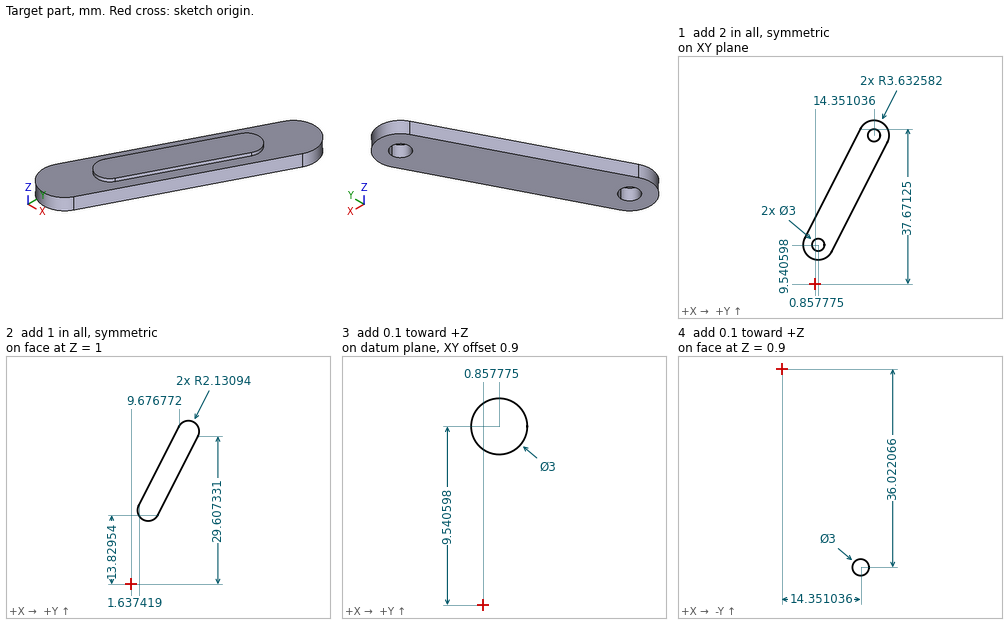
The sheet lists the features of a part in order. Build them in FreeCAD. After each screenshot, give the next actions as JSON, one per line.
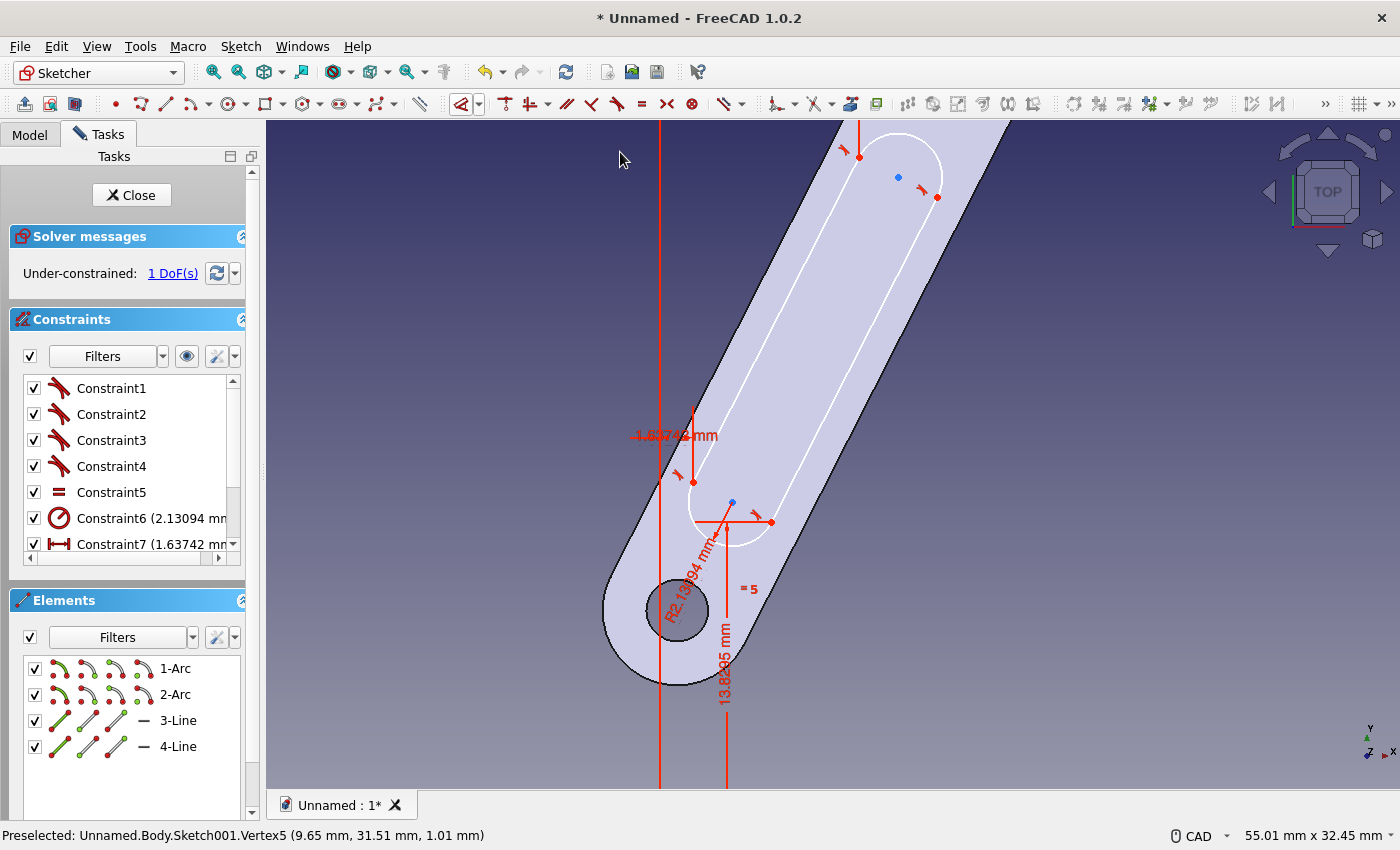
{"action": "left_click", "coordinate": [937, 197]}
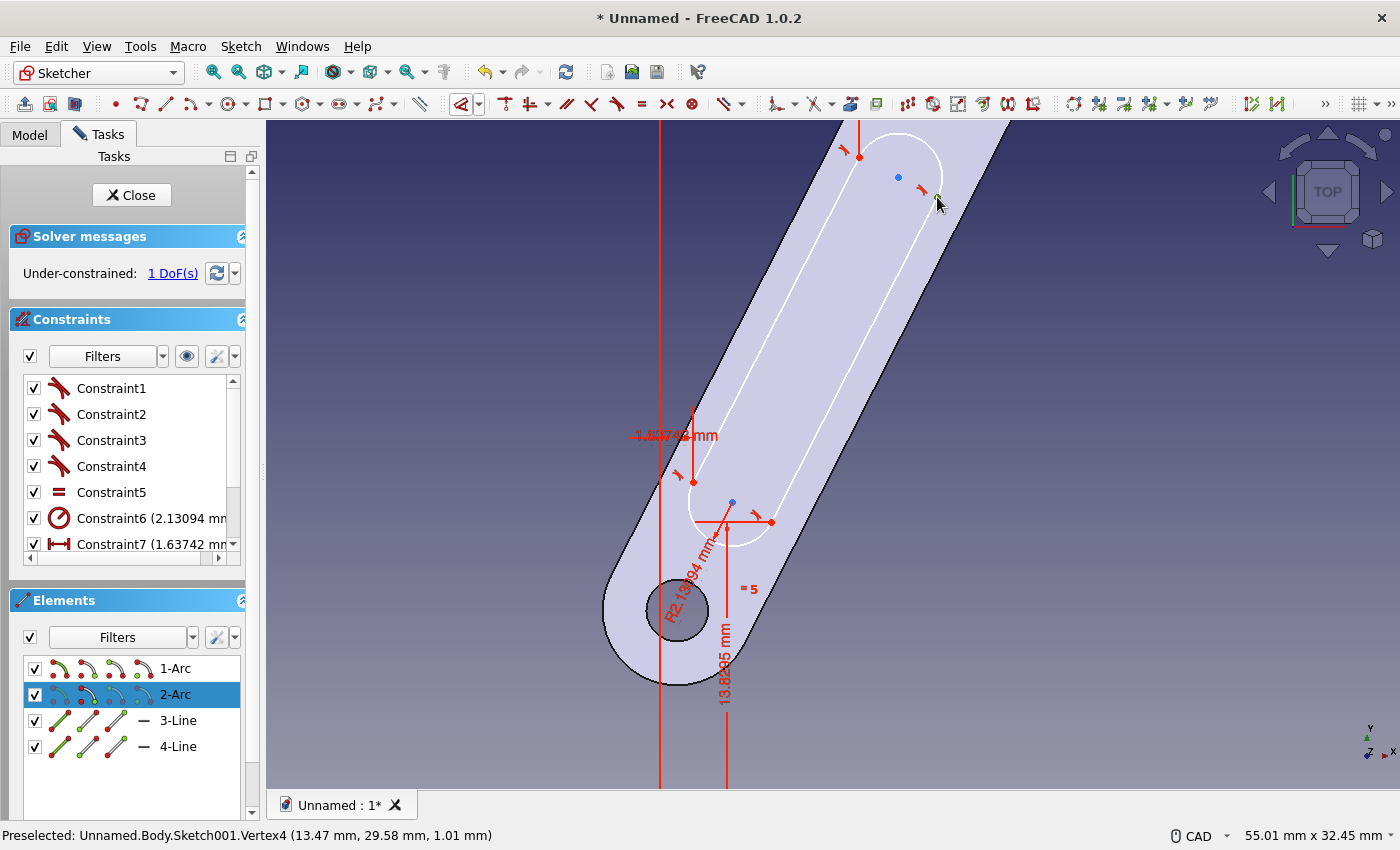
{"action": "key", "text": "i"}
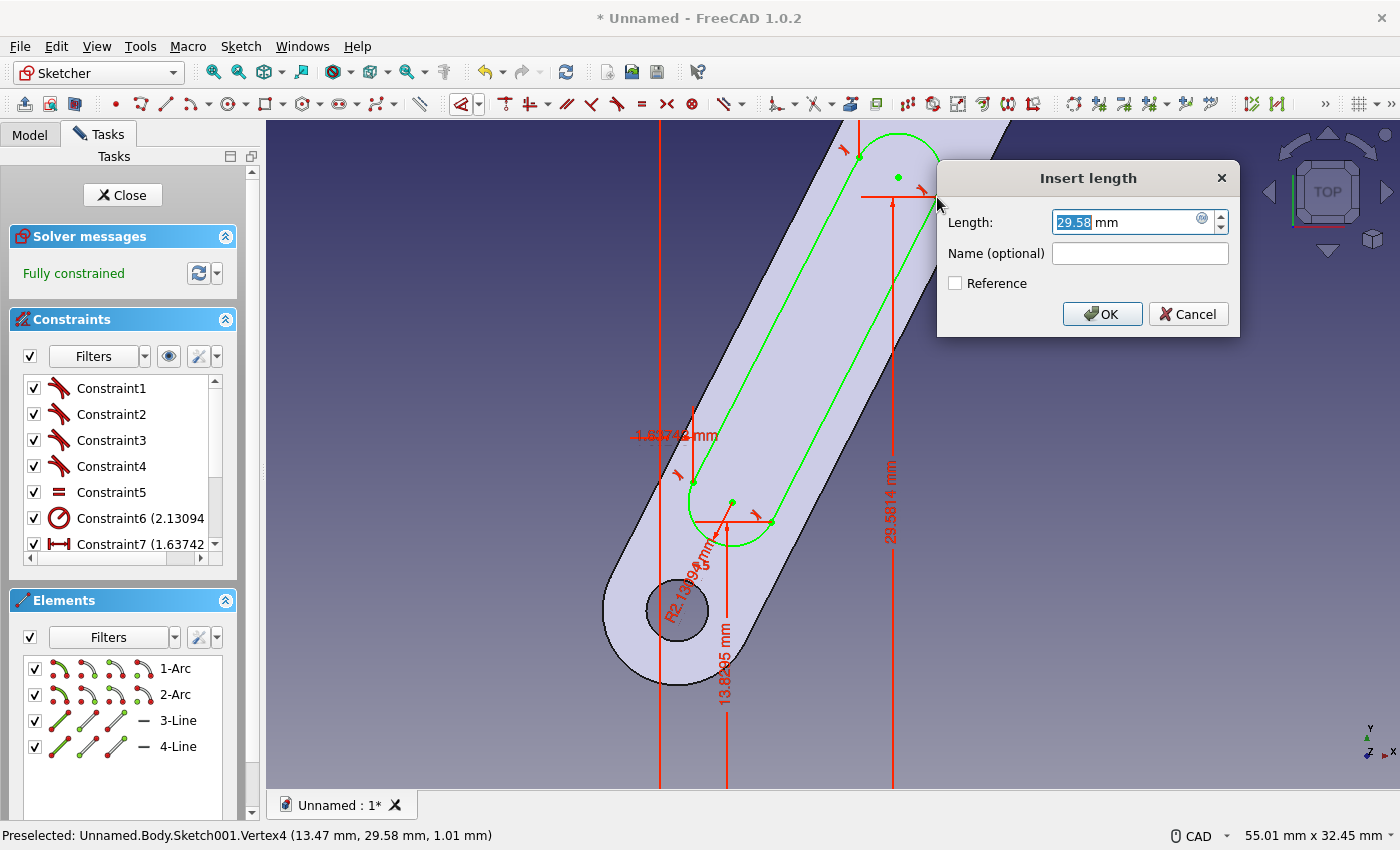
{"action": "type", "text": "29.607331"}
{"action": "key", "text": "Return"}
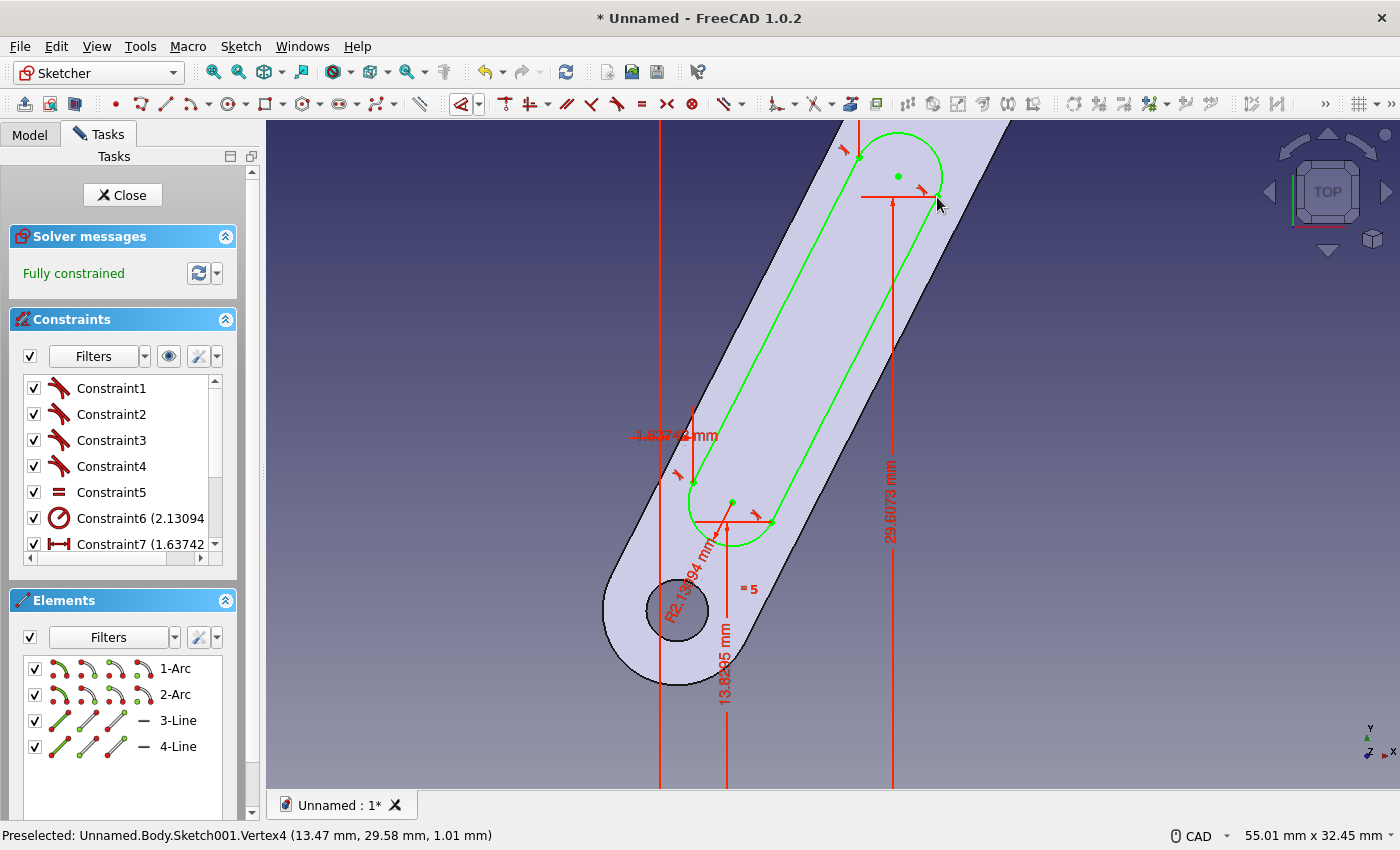
{"action": "left_click", "coordinate": [123, 195]}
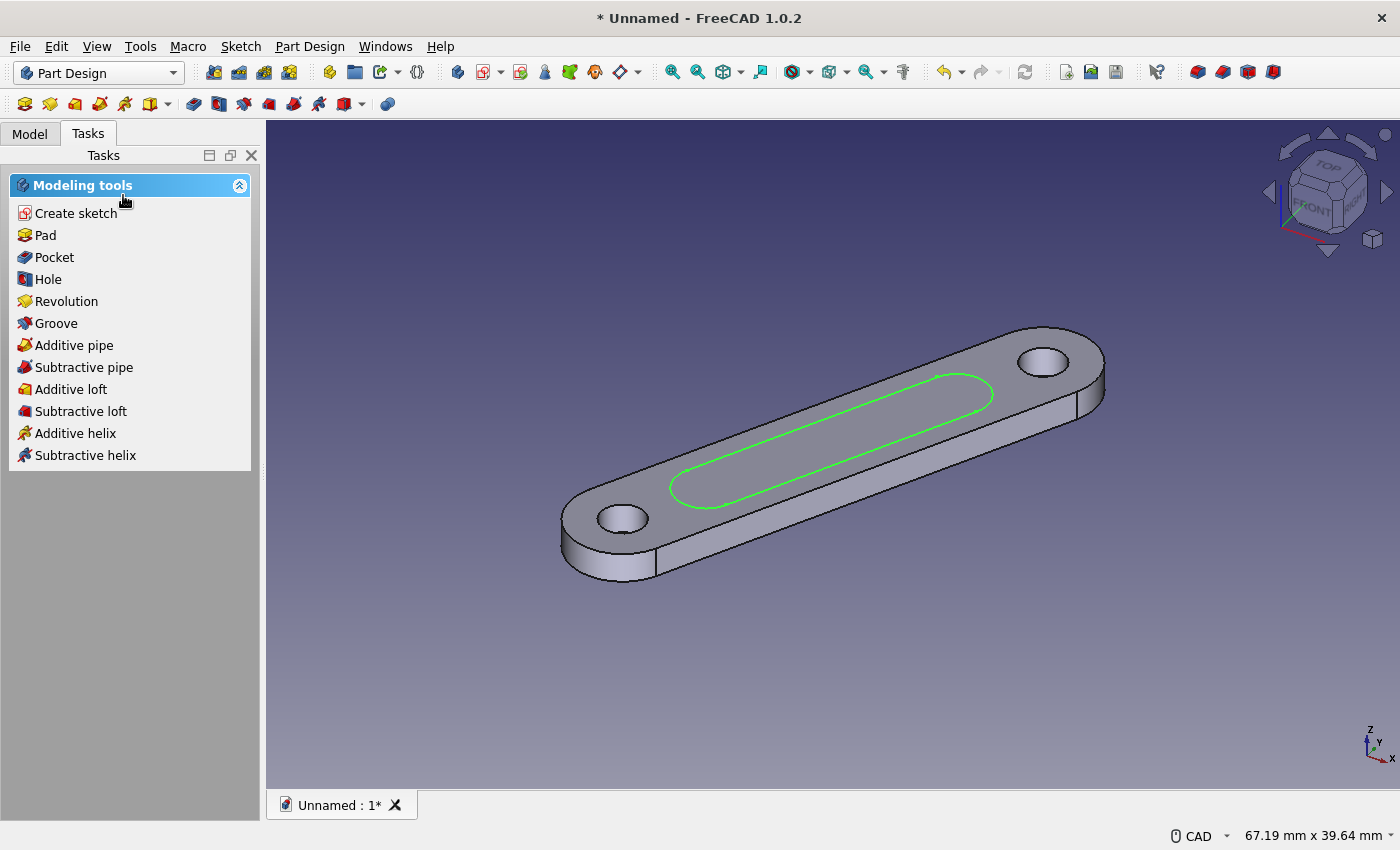
{"action": "left_click", "coordinate": [25, 104]}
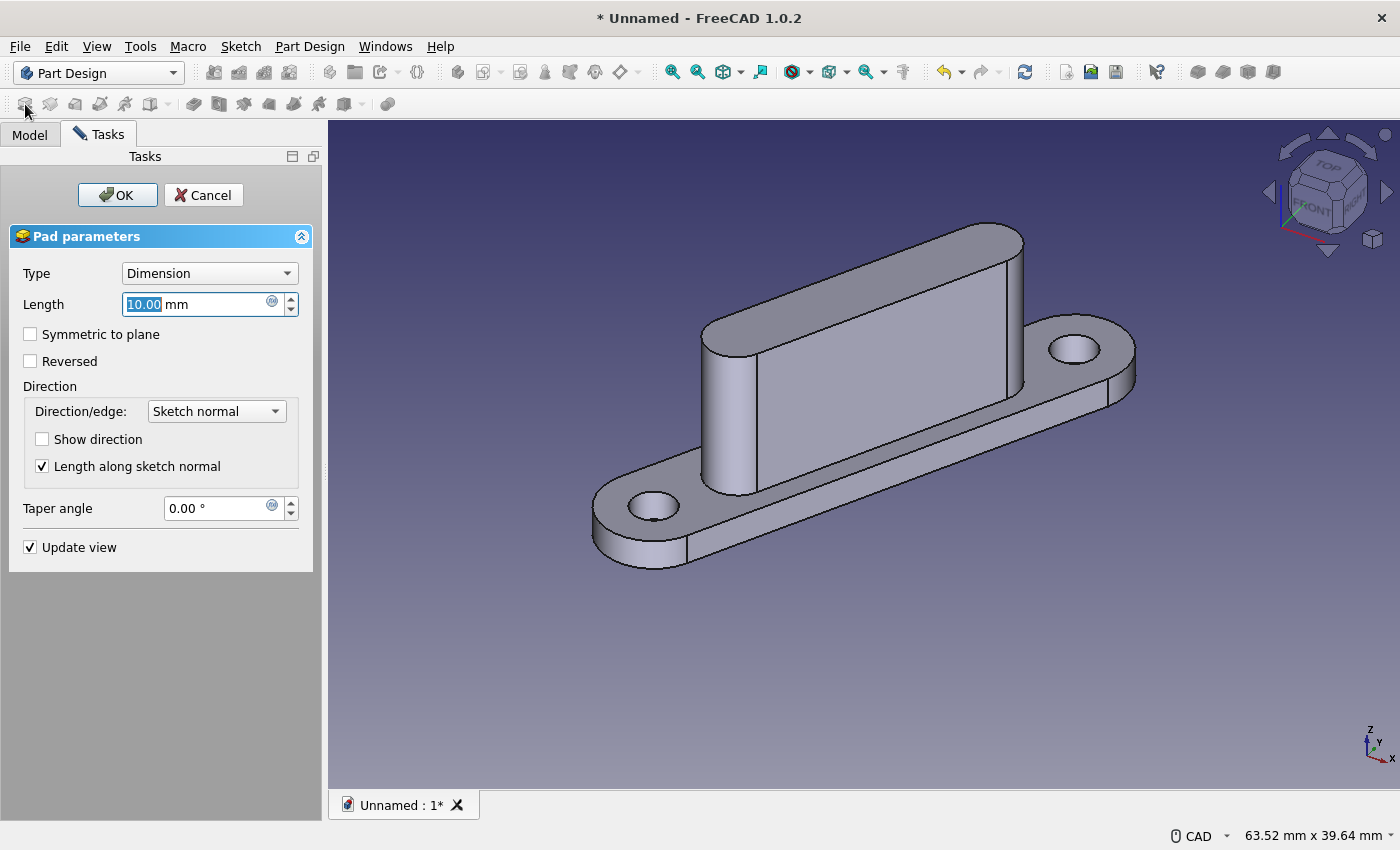
{"action": "type", "text": "1"}
{"action": "key", "text": "Tab"}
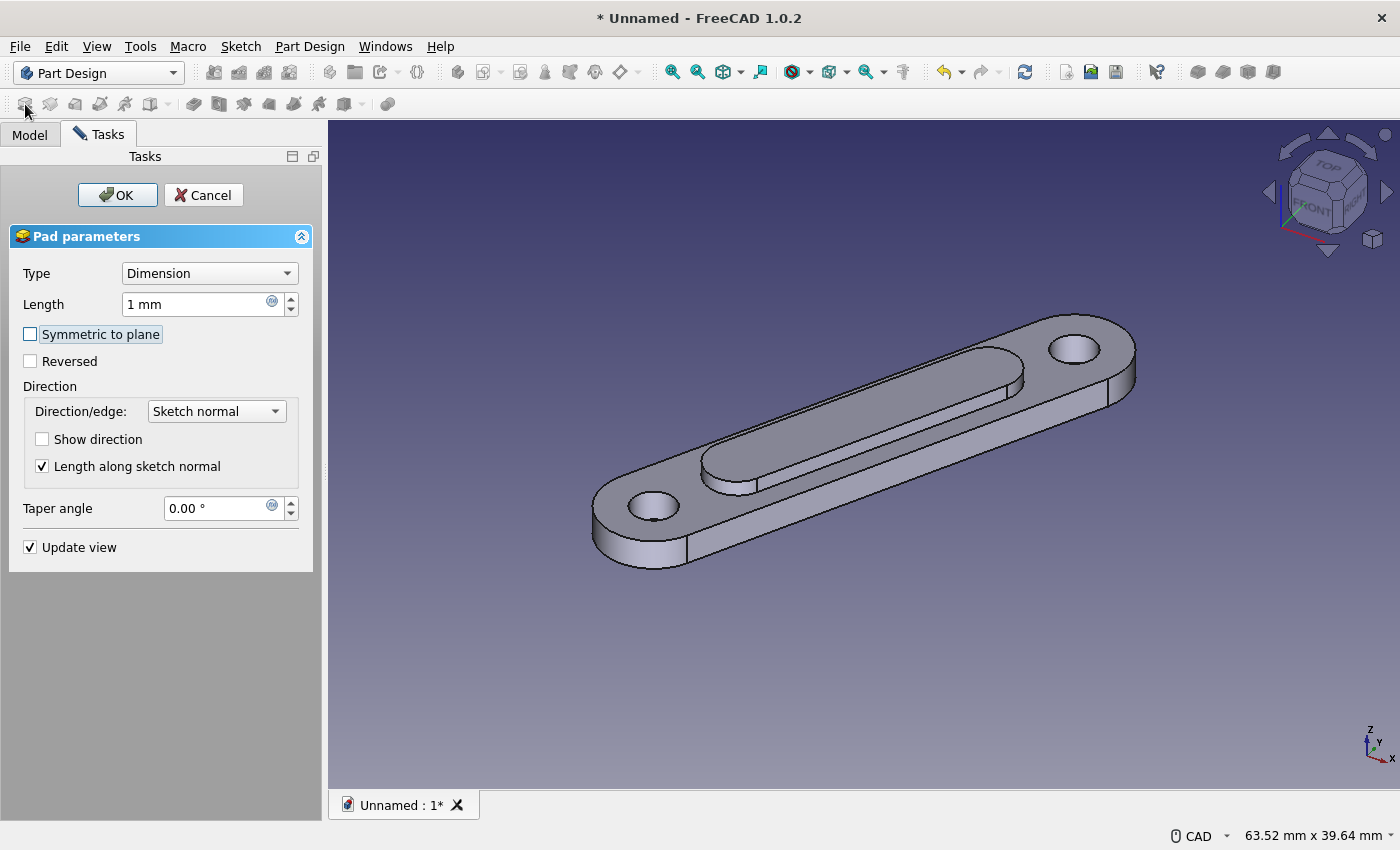
{"action": "left_click", "coordinate": [31, 334]}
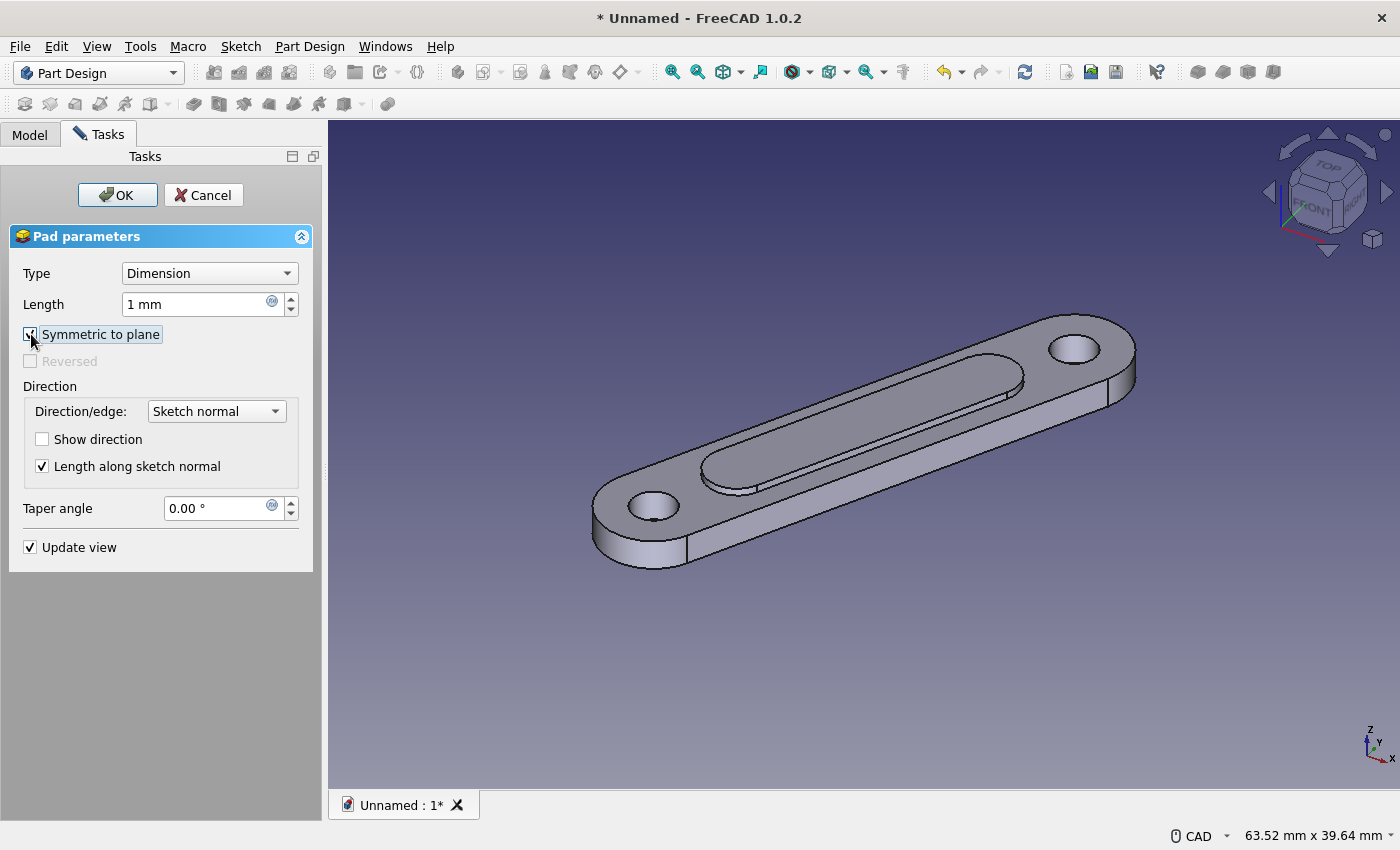
{"action": "left_click", "coordinate": [118, 195]}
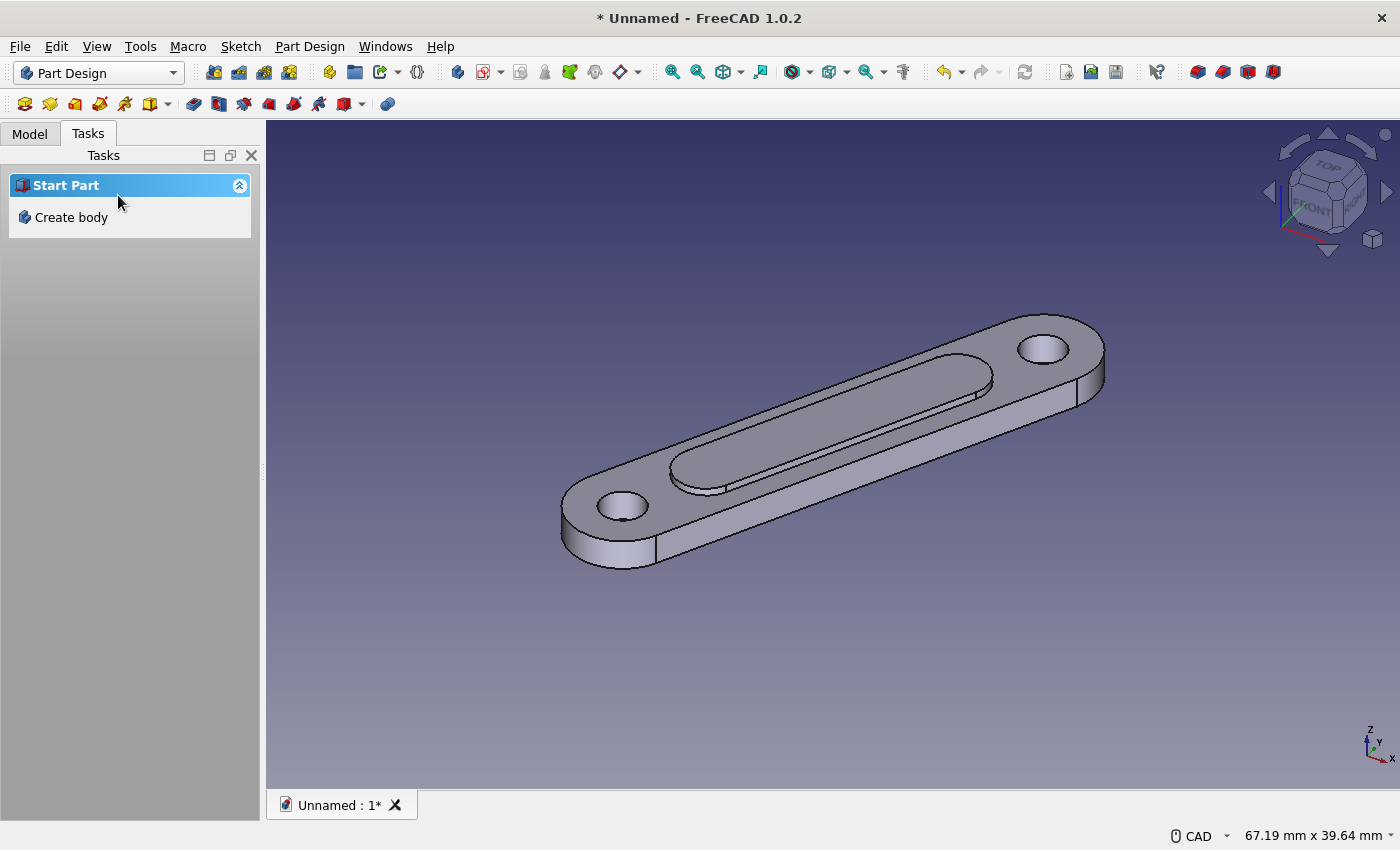
{"action": "left_click", "coordinate": [30, 134]}